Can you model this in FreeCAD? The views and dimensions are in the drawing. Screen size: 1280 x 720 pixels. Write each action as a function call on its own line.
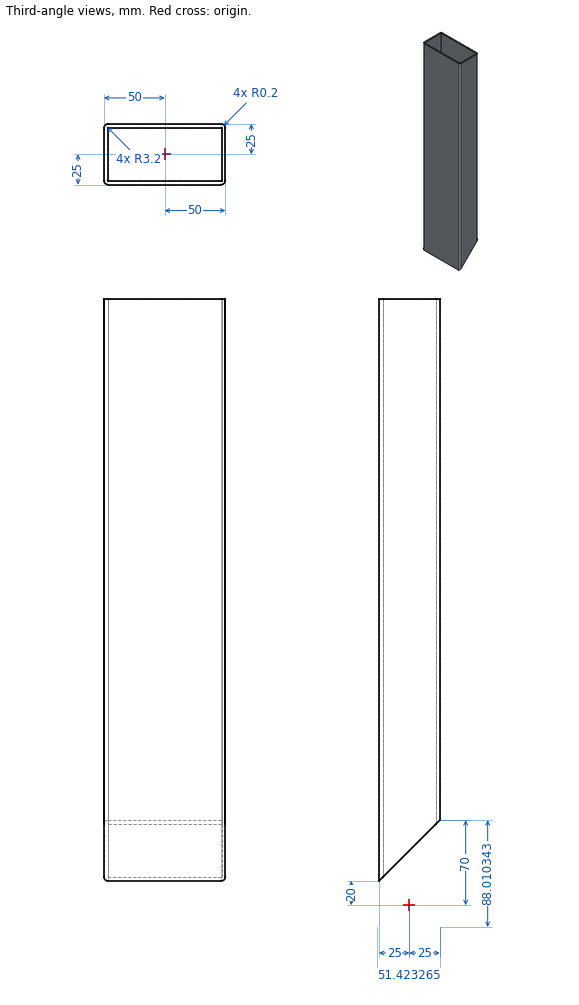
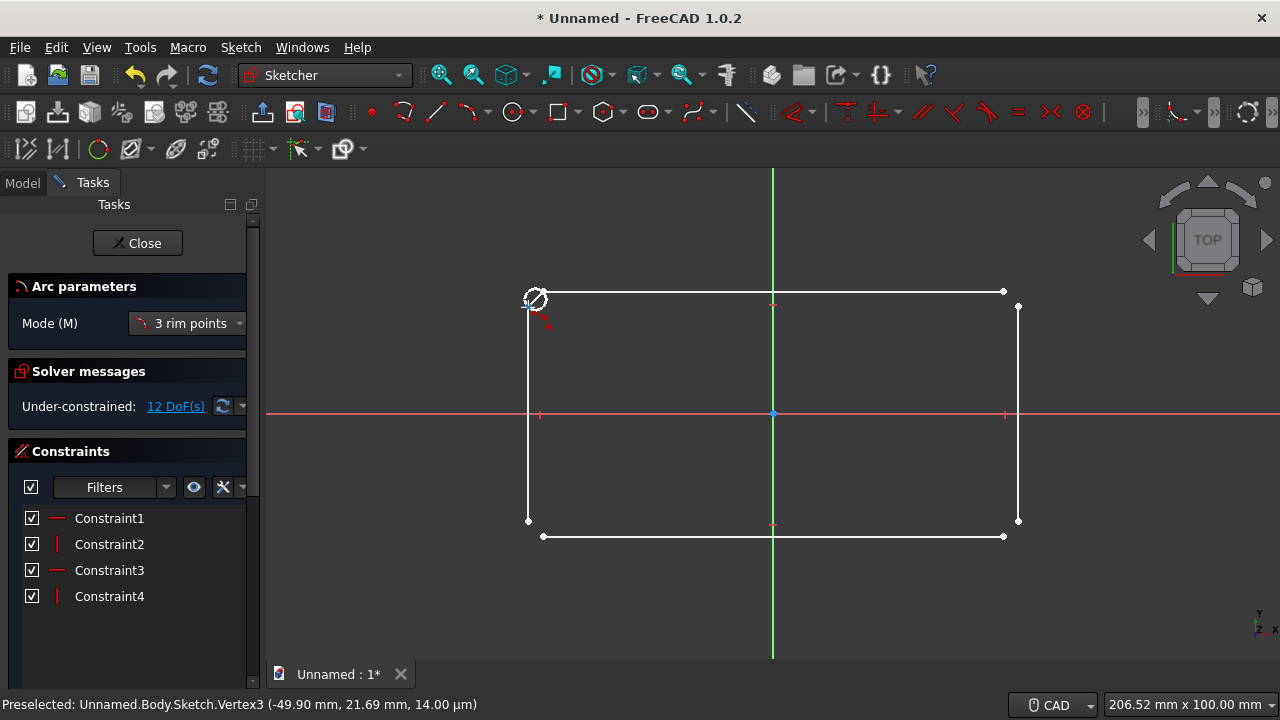
scroll(532, 295, up, 7)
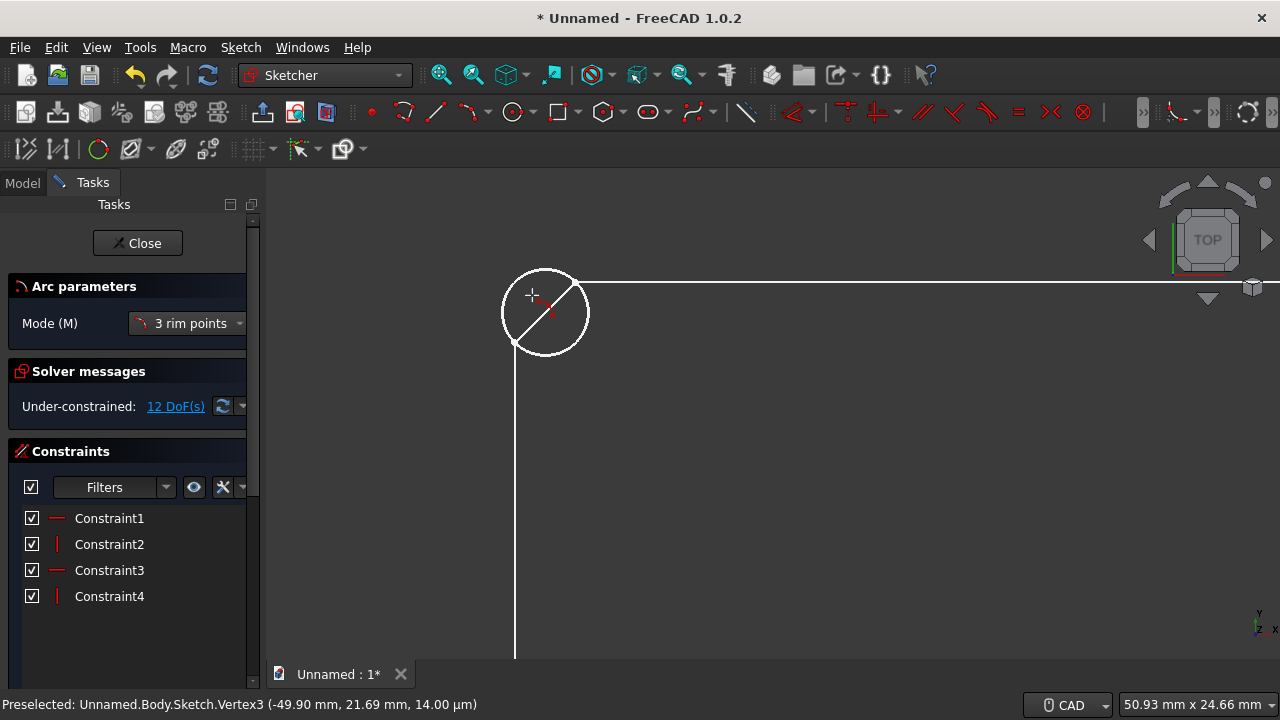
click(532, 296)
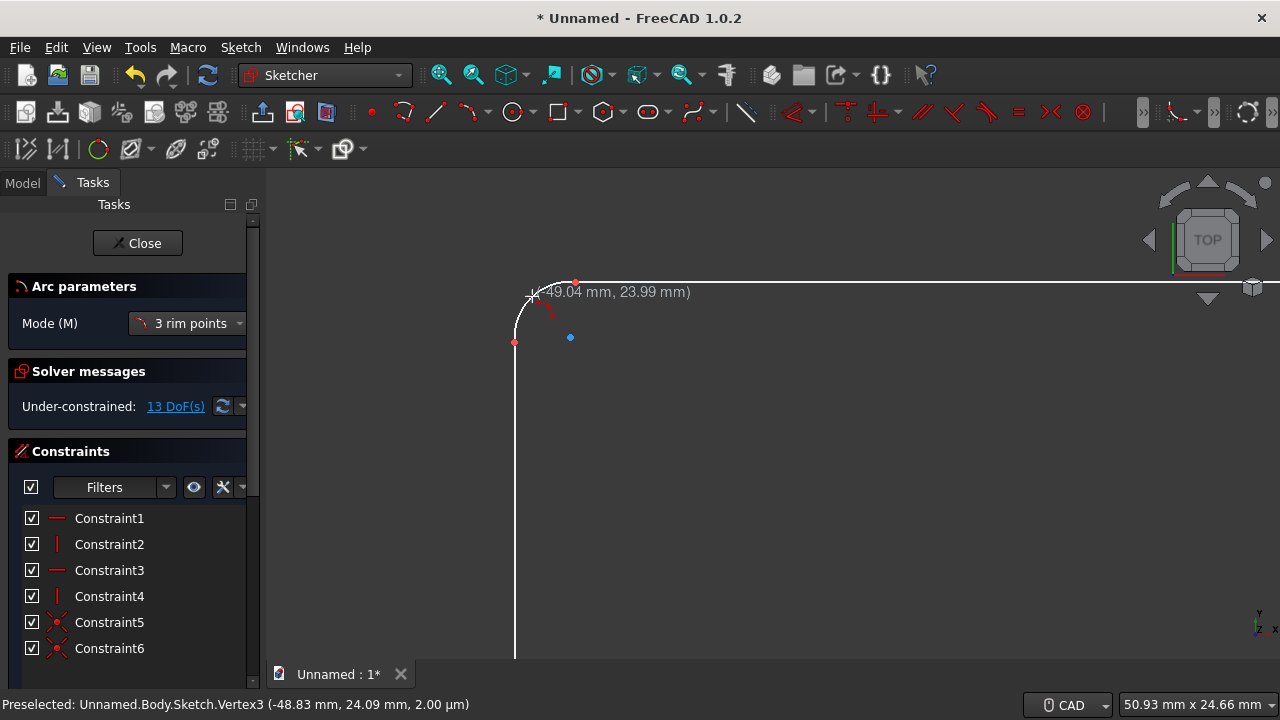
scroll(358, 258, down, 6)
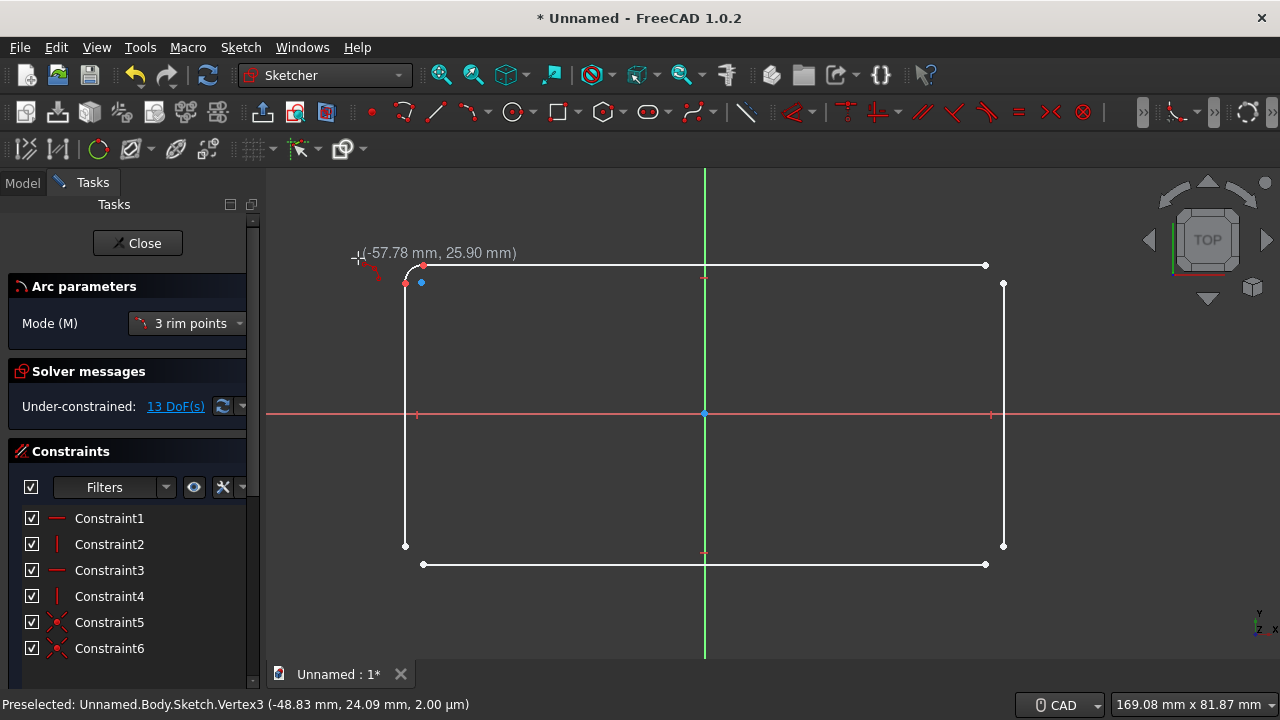
click(405, 546)
click(424, 565)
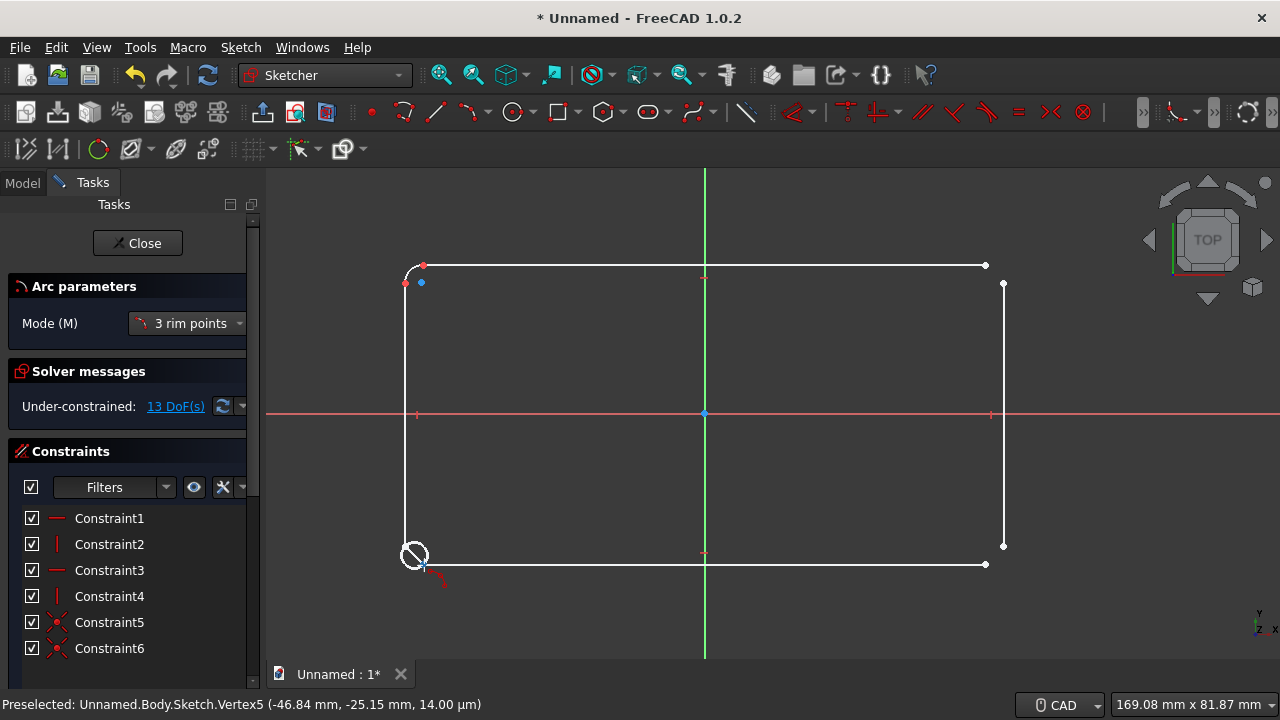
scroll(410, 558, up, 6)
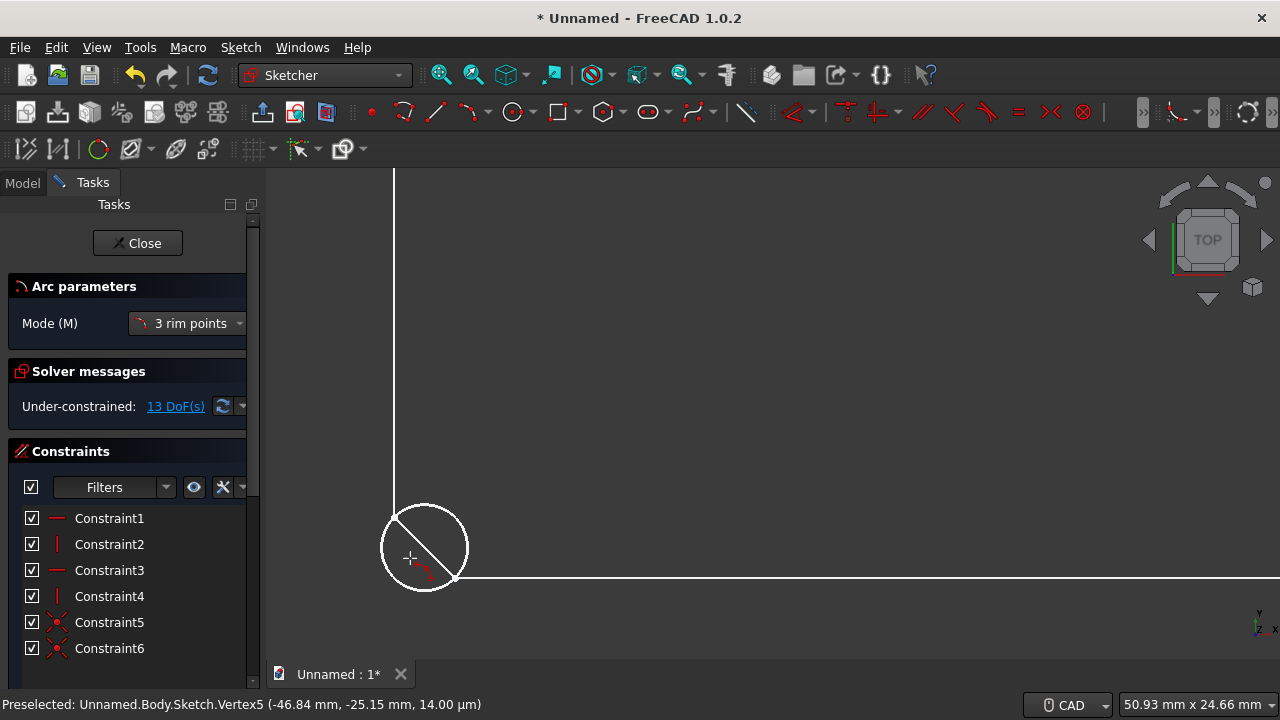
click(411, 556)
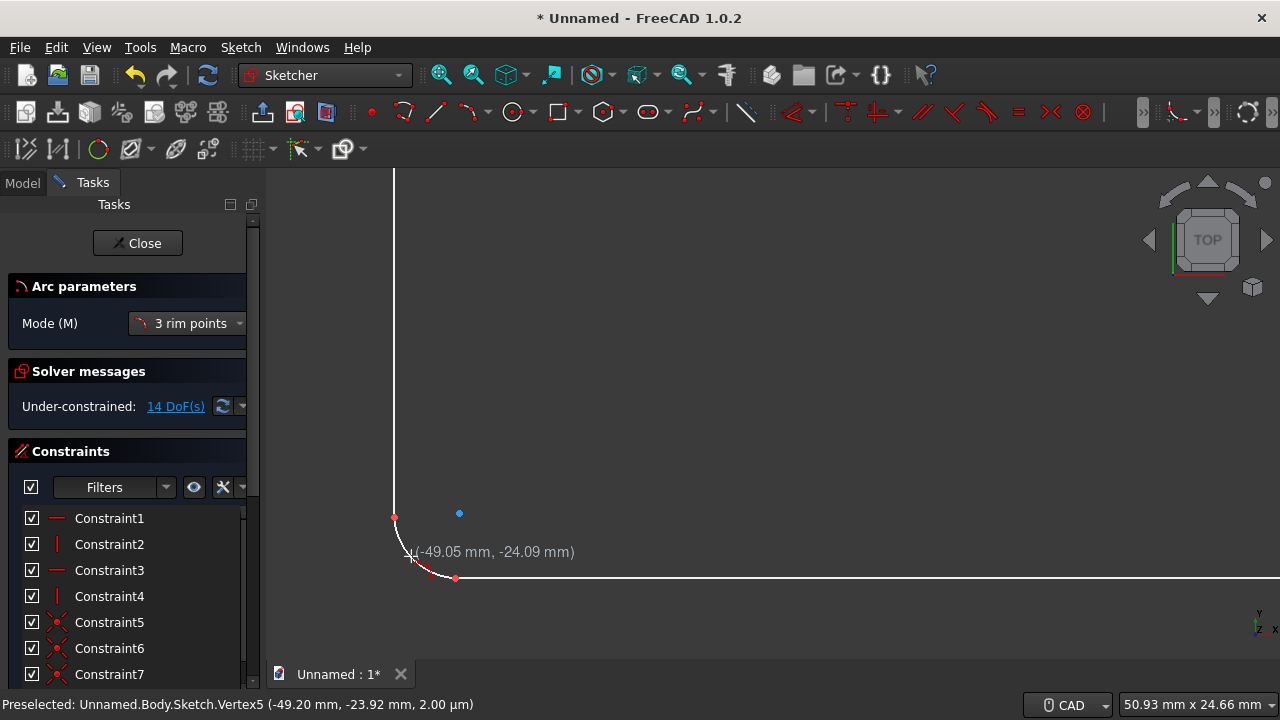
scroll(410, 558, down, 6)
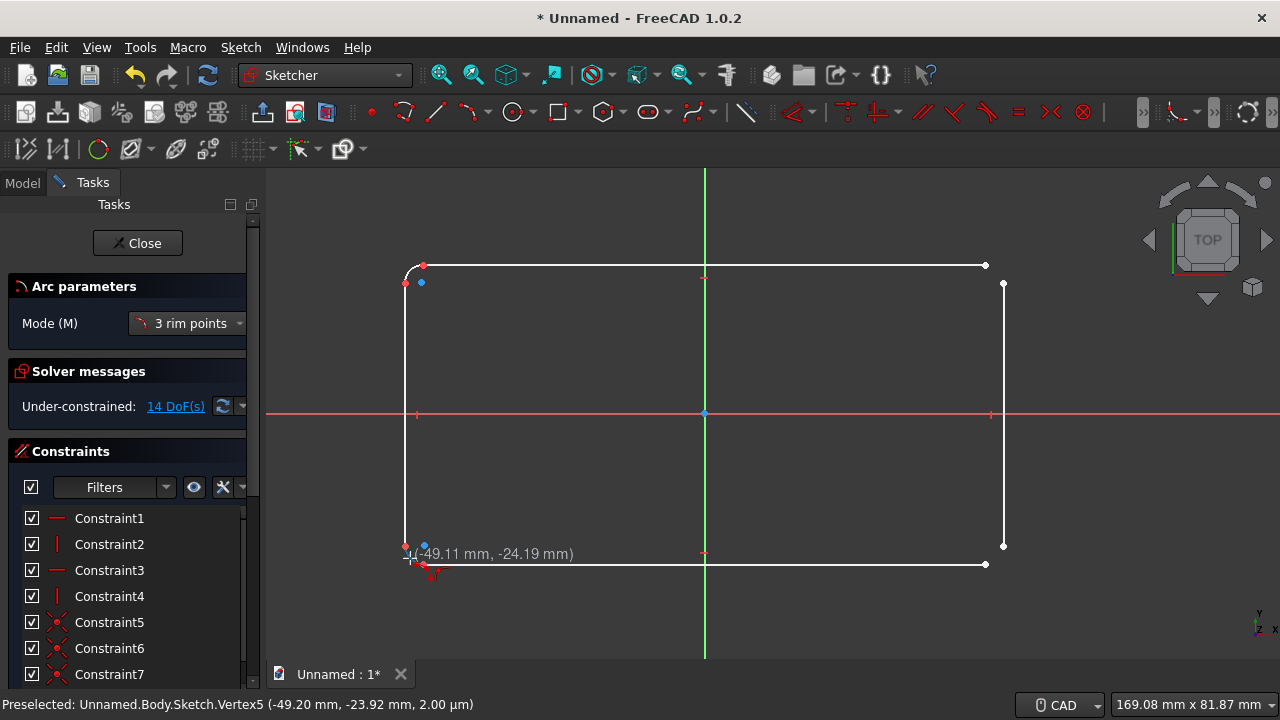
click(986, 565)
click(1004, 546)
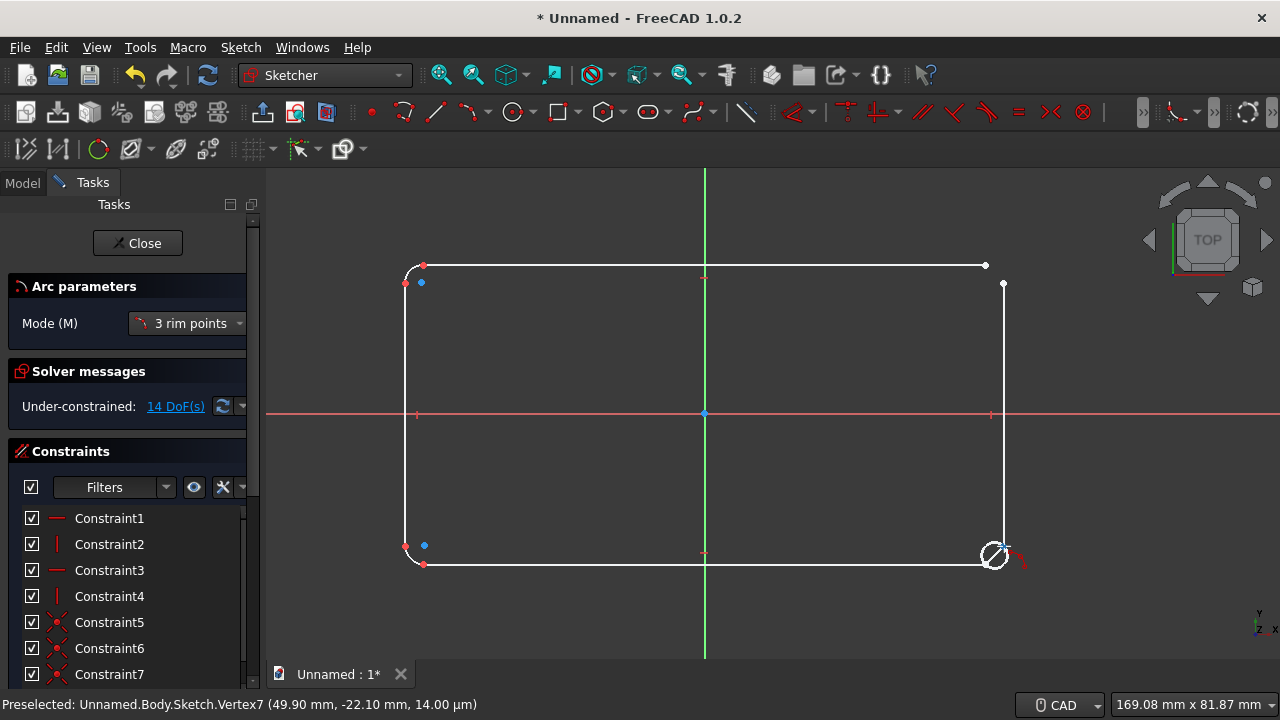
scroll(999, 558, up, 6)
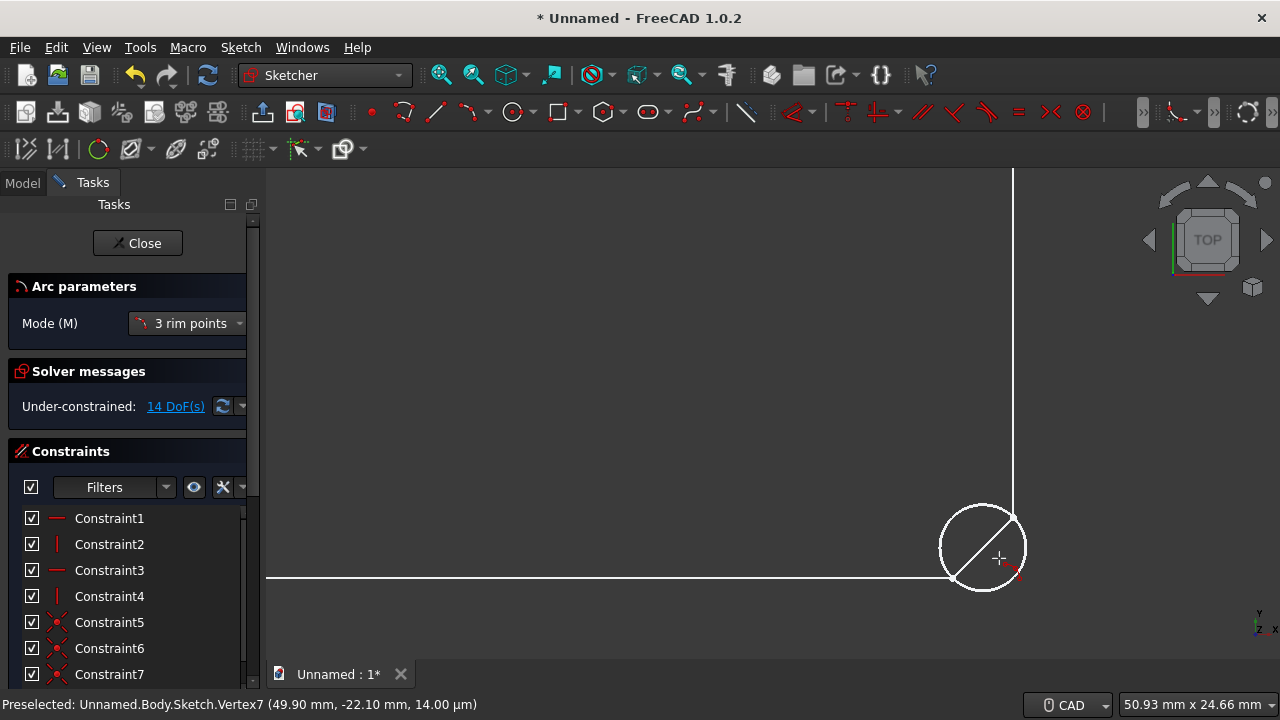
click(997, 556)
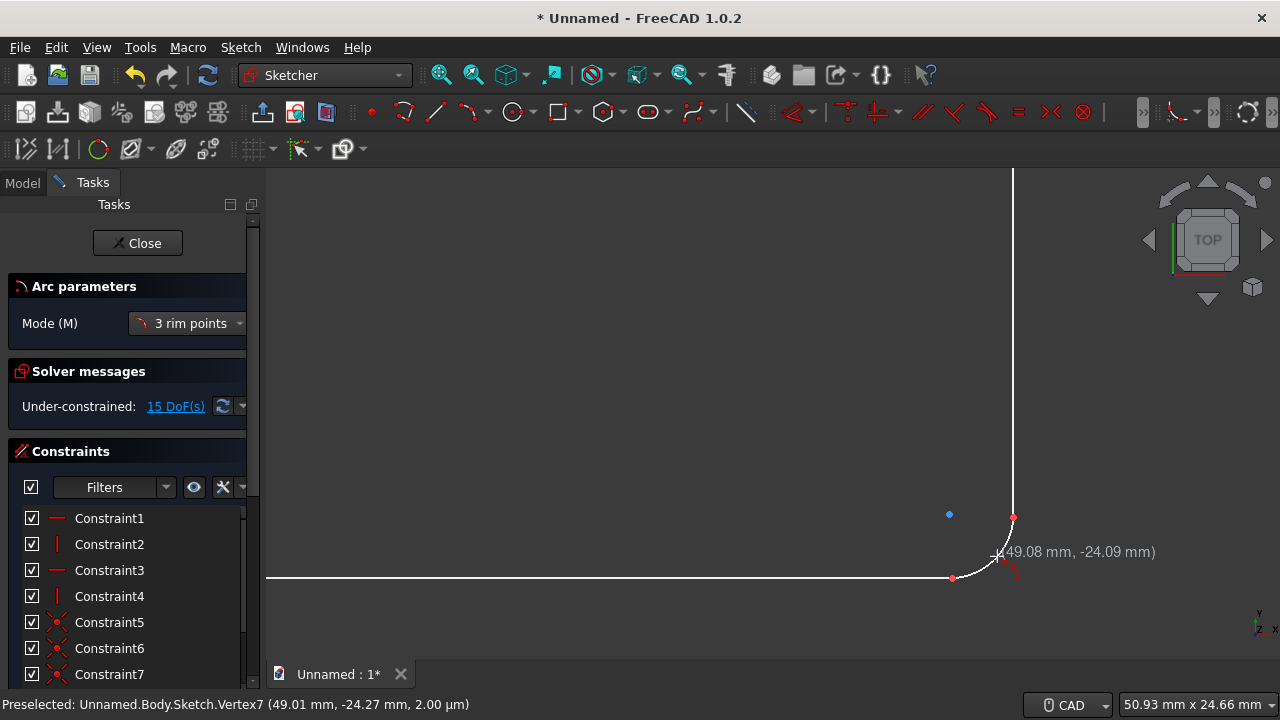
scroll(1000, 558, down, 6)